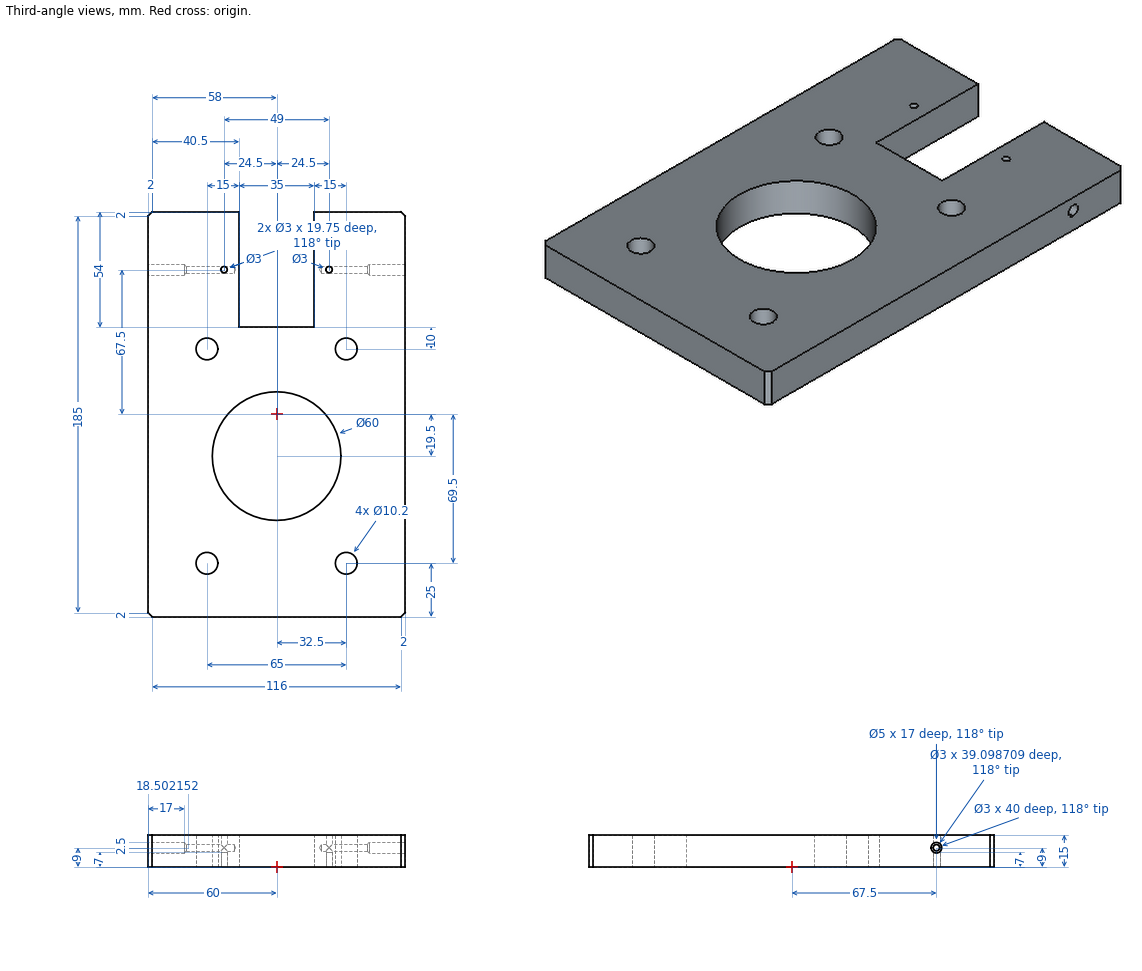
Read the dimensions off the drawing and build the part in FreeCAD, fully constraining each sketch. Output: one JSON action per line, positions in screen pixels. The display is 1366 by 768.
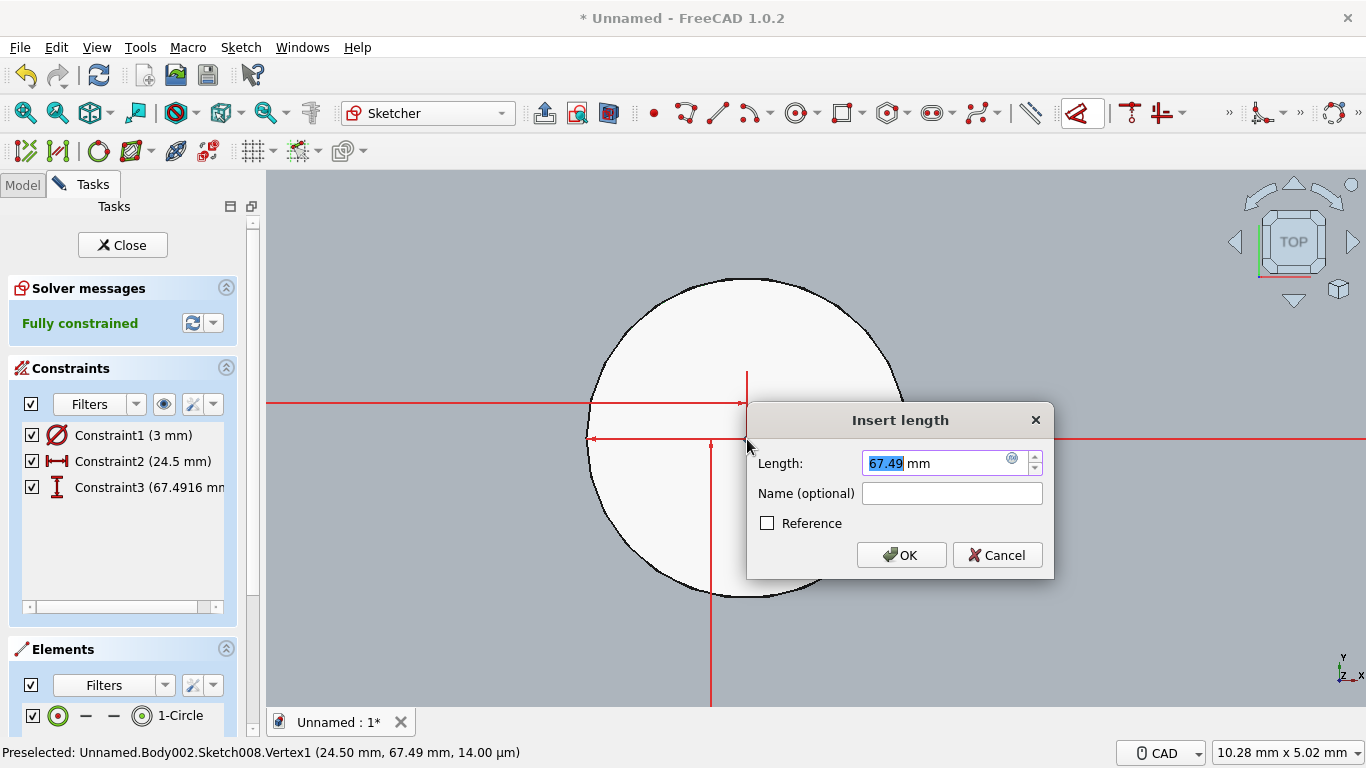
{"action": "type", "text": "67.5"}
{"action": "key", "text": "Return"}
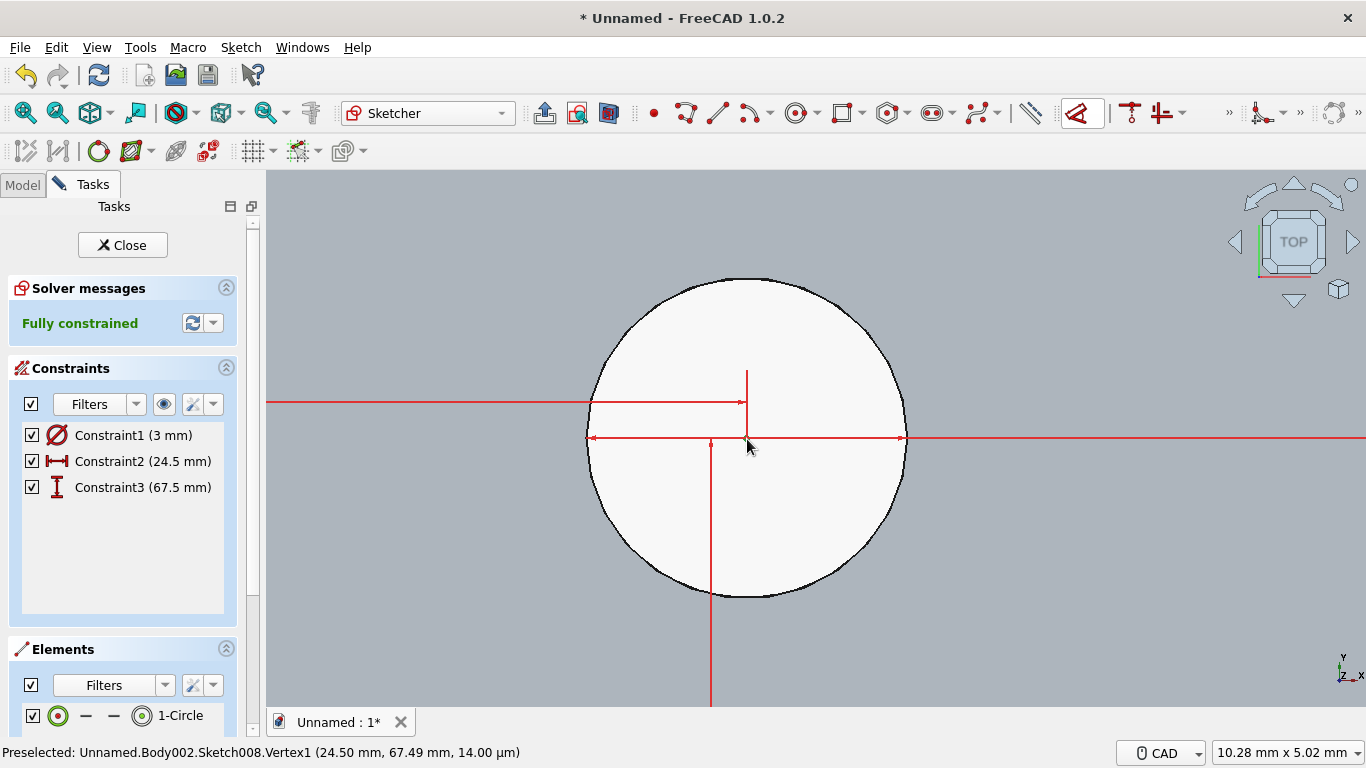
{"action": "left_click", "coordinate": [123, 245]}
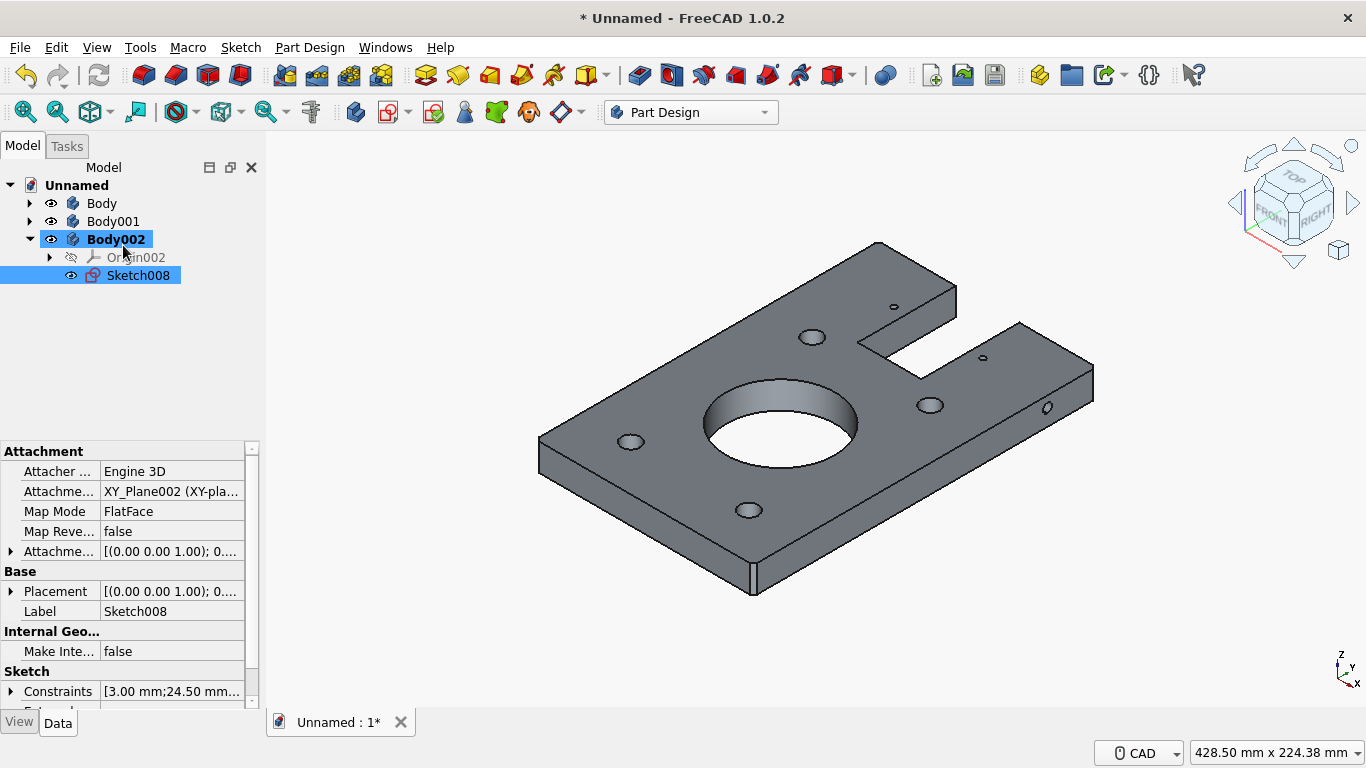
{"action": "left_click", "coordinate": [426, 76]}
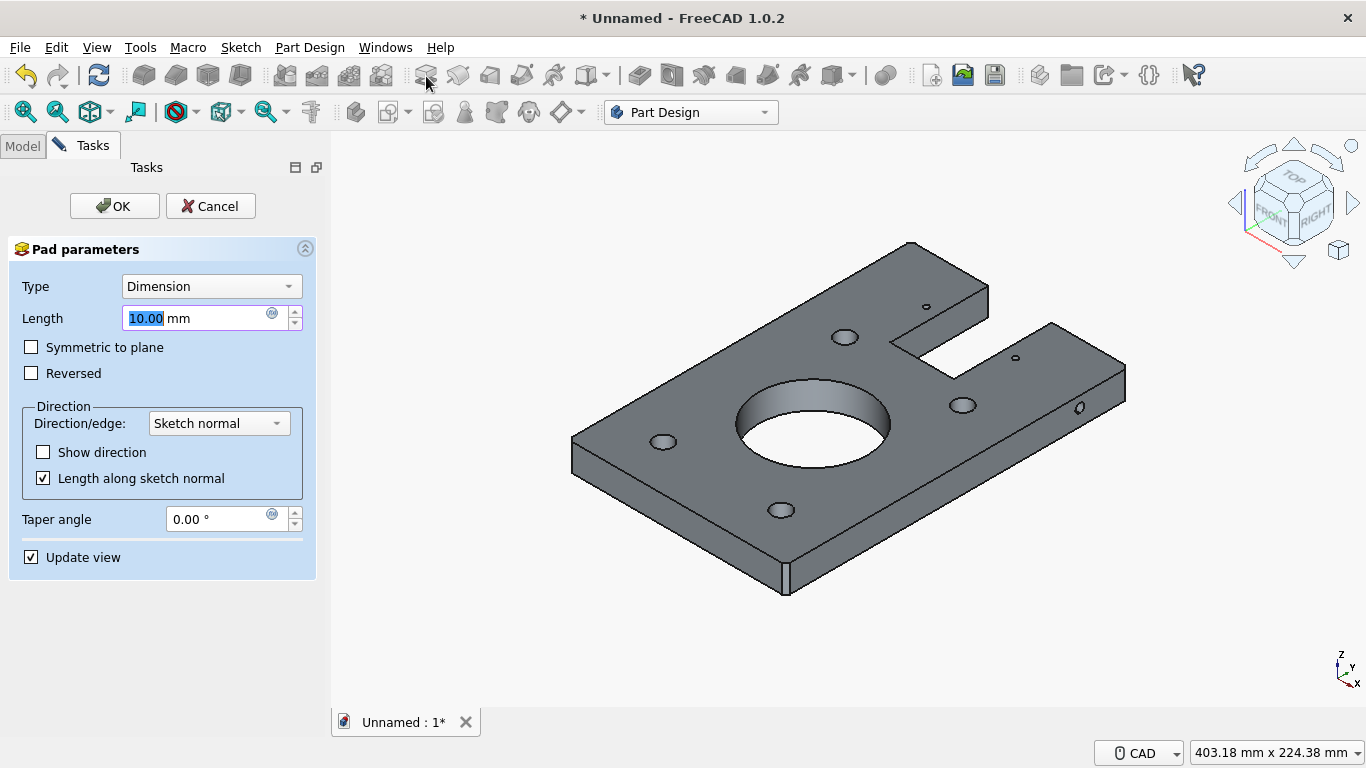
{"action": "type", "text": "7"}
{"action": "key", "text": "Tab"}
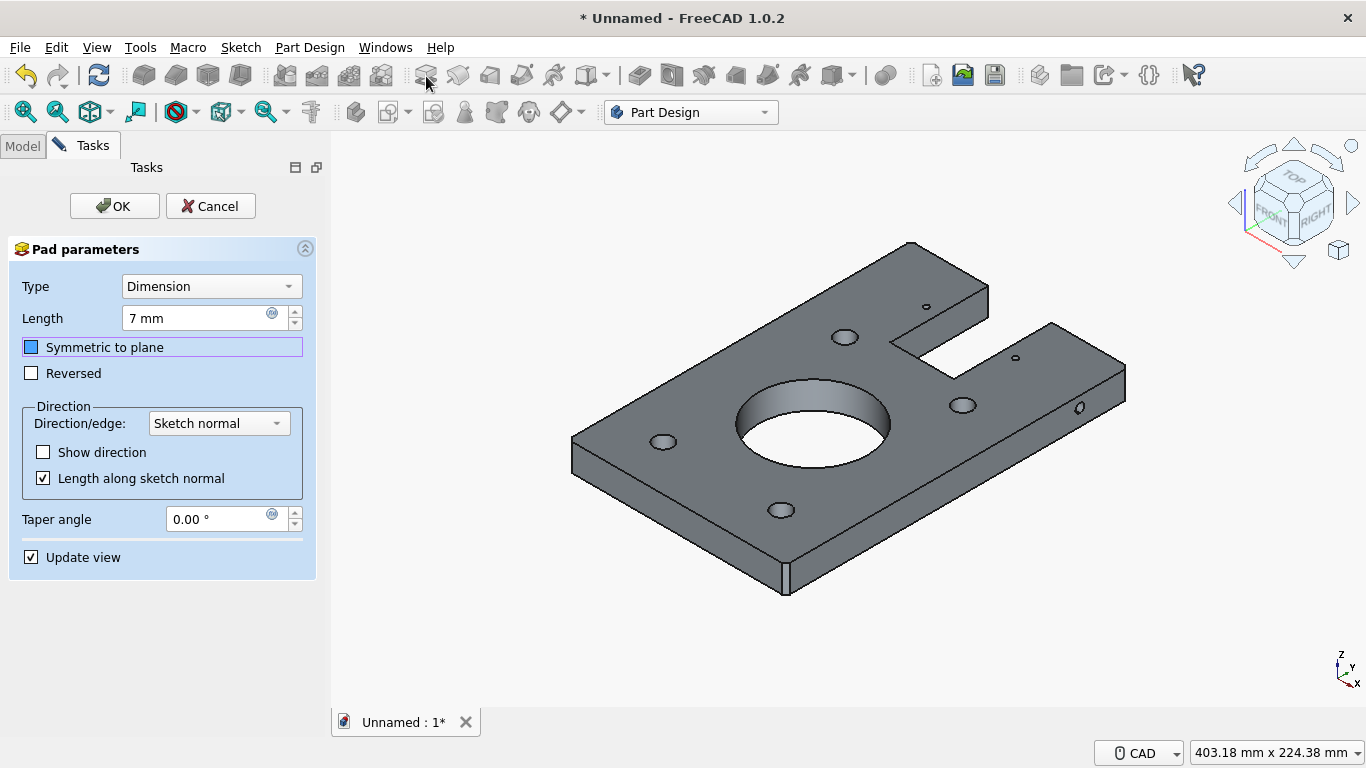
{"action": "left_click", "coordinate": [115, 206]}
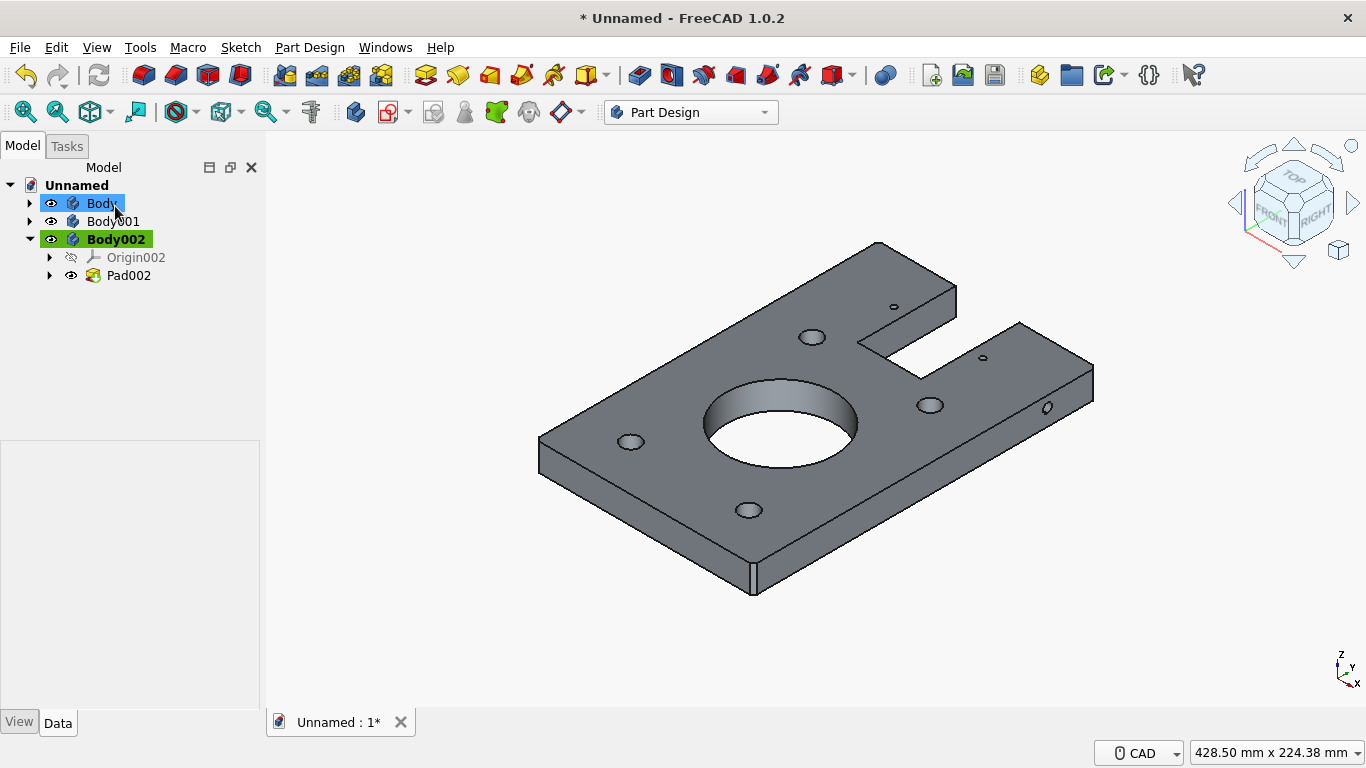
{"action": "left_click", "coordinate": [26, 112]}